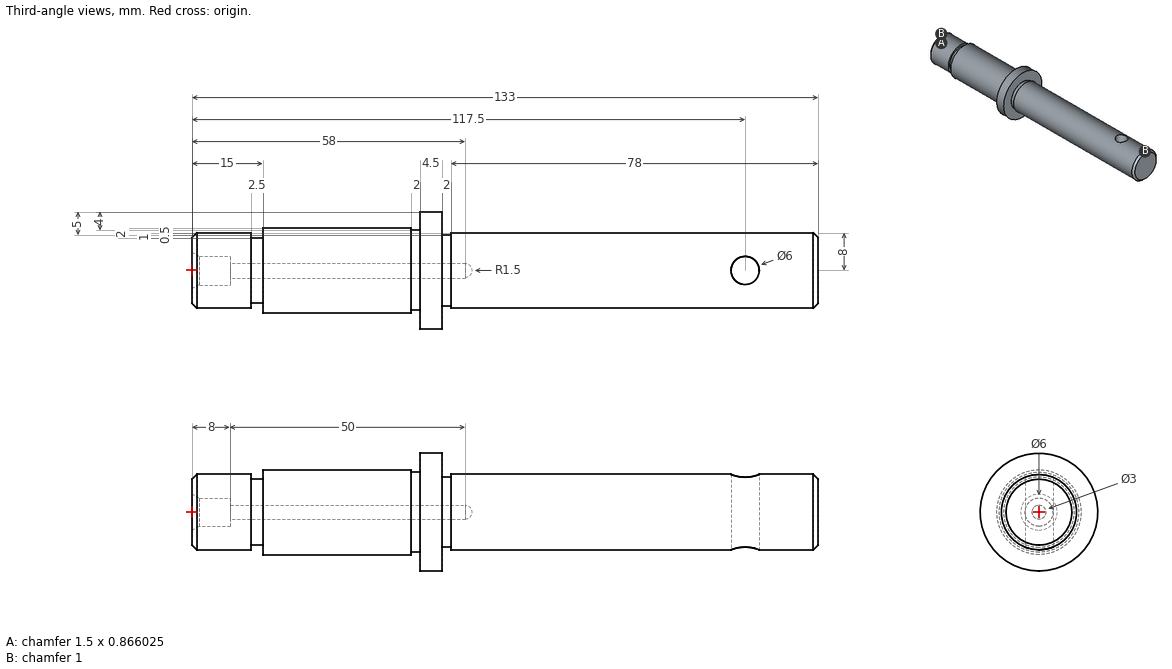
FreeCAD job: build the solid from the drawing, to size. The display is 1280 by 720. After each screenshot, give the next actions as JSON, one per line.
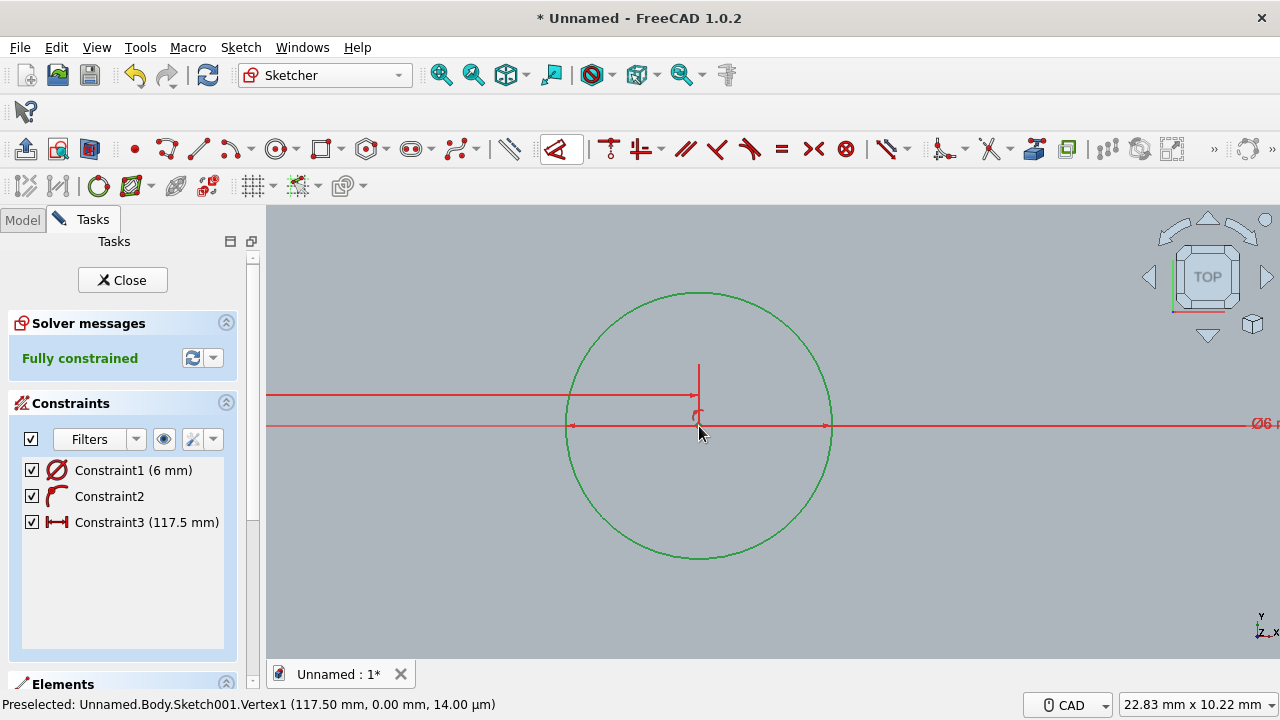
{"action": "left_click", "coordinate": [123, 280]}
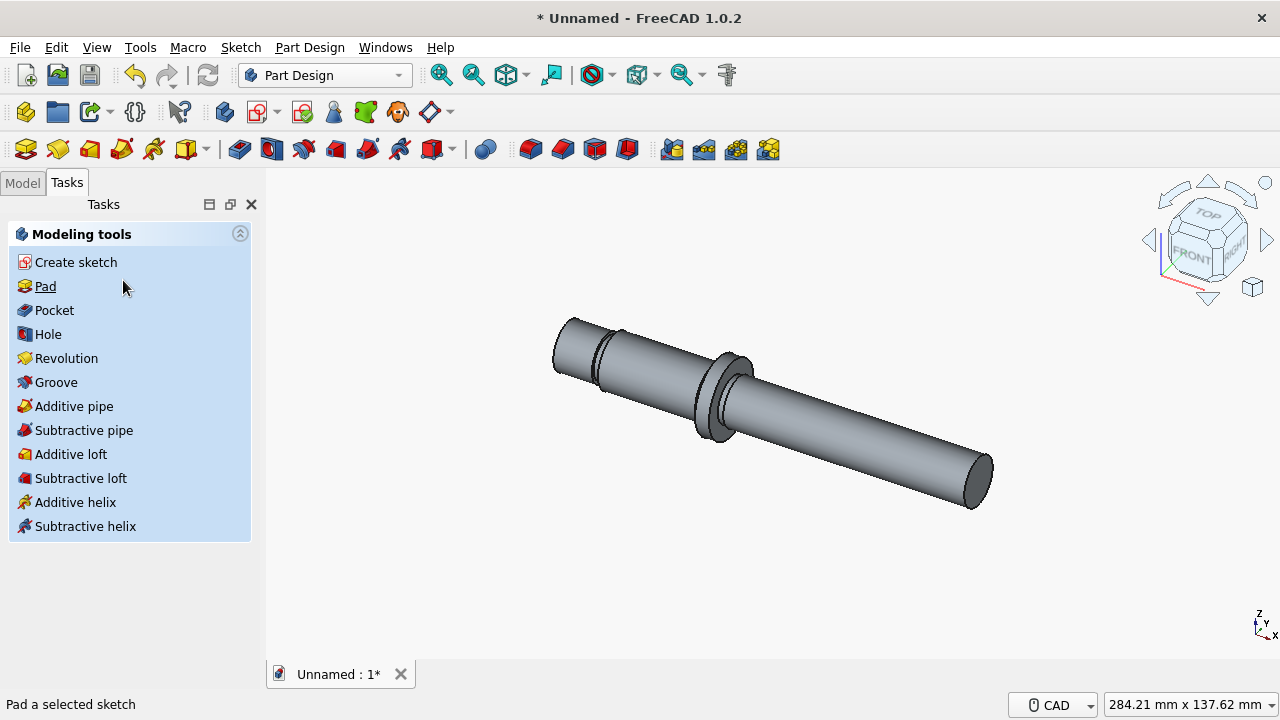
{"action": "left_click", "coordinate": [240, 150]}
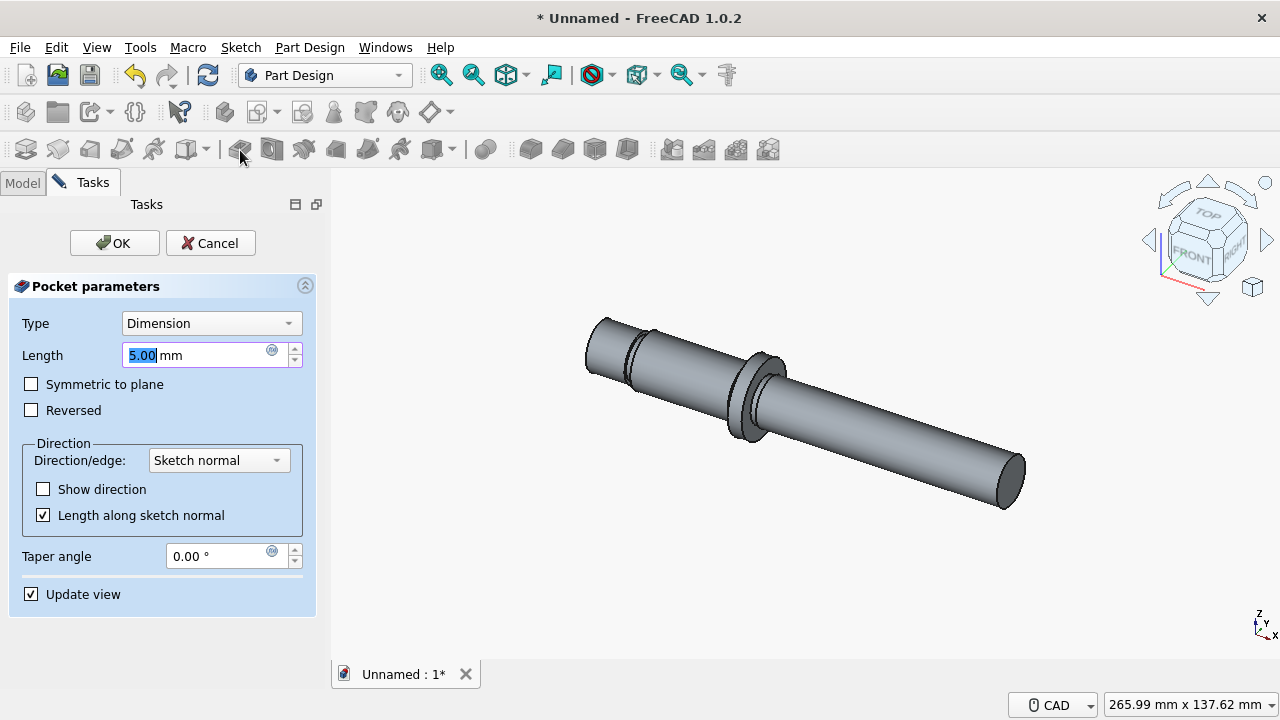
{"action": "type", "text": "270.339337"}
{"action": "key", "text": "Tab"}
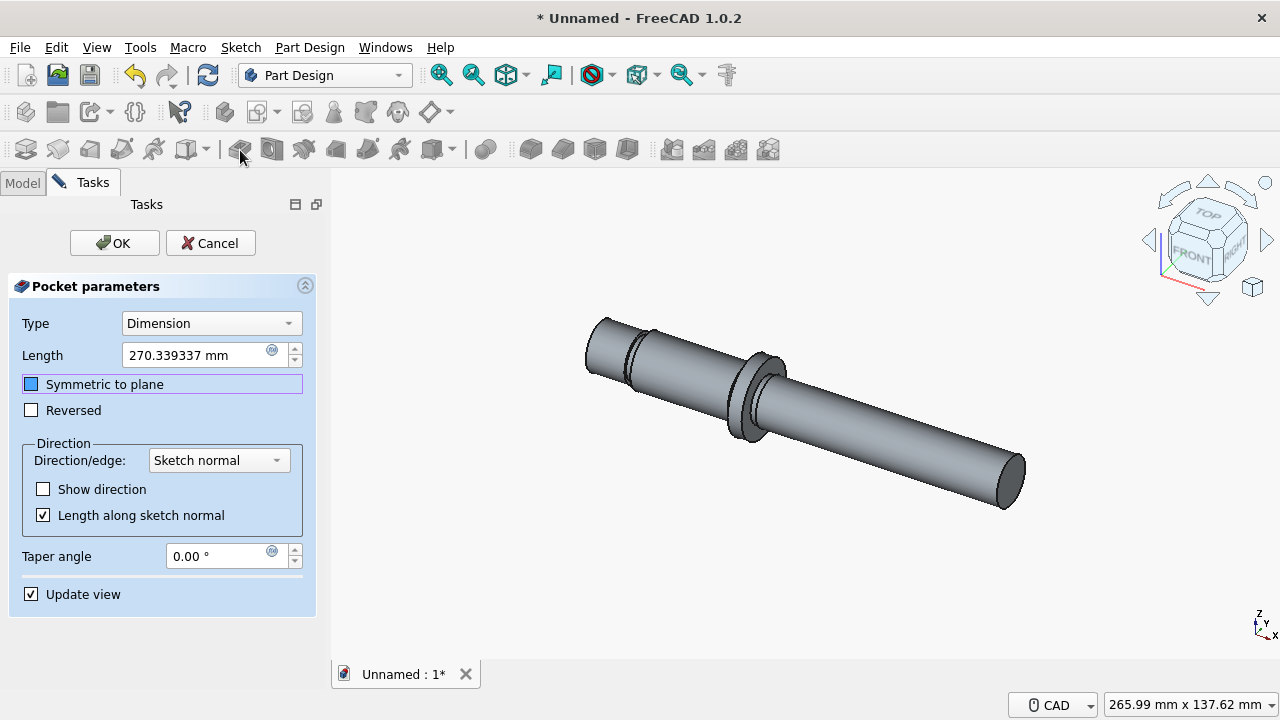
{"action": "left_click", "coordinate": [30, 384]}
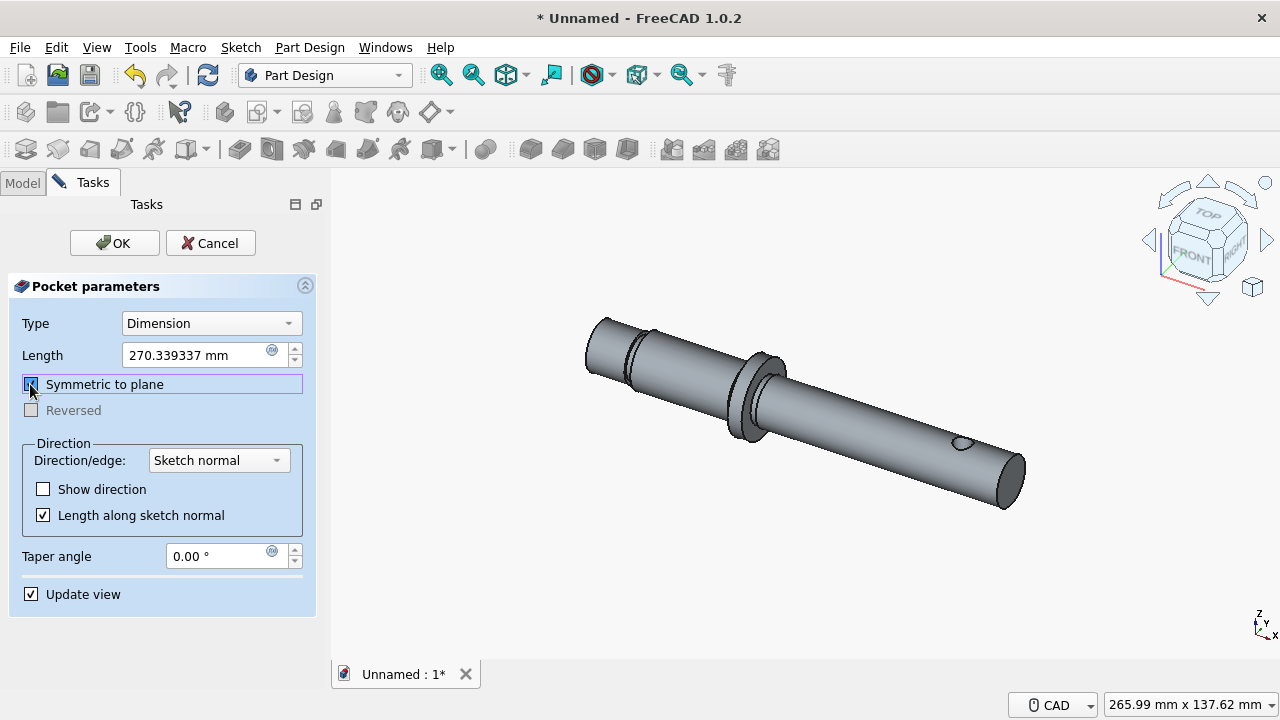
{"action": "left_click", "coordinate": [115, 243]}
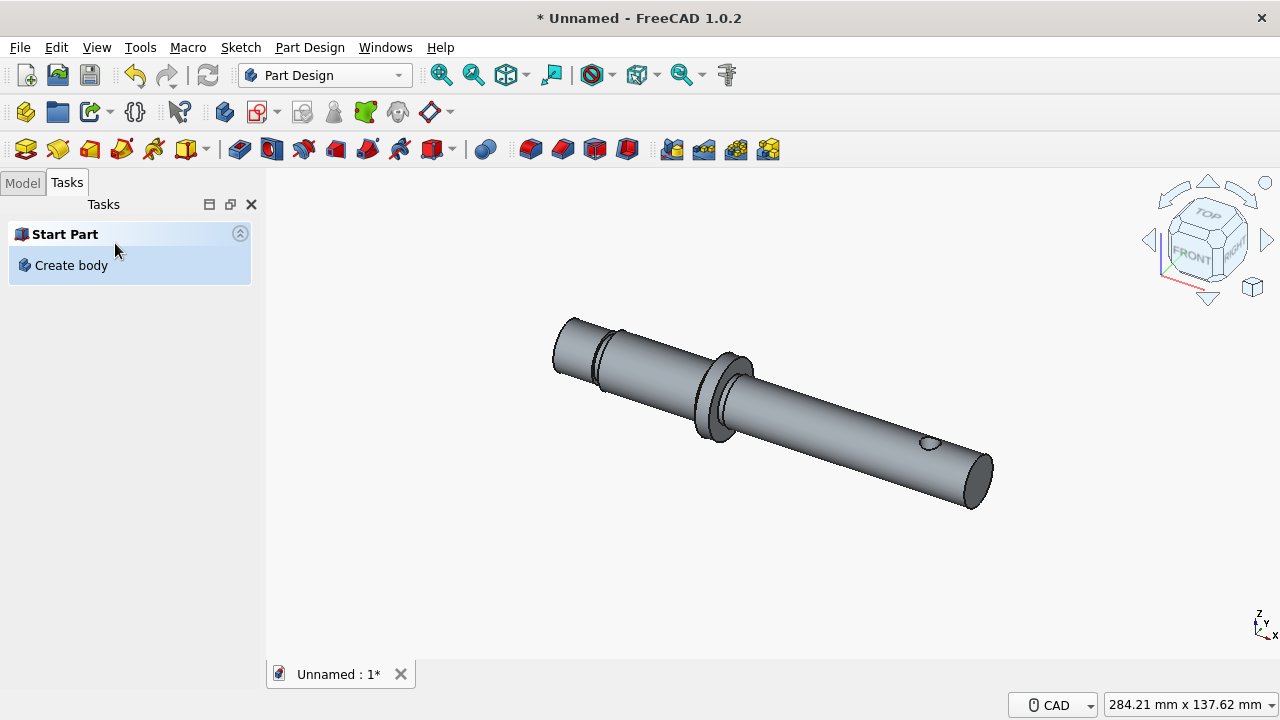
{"action": "key", "text": "6"}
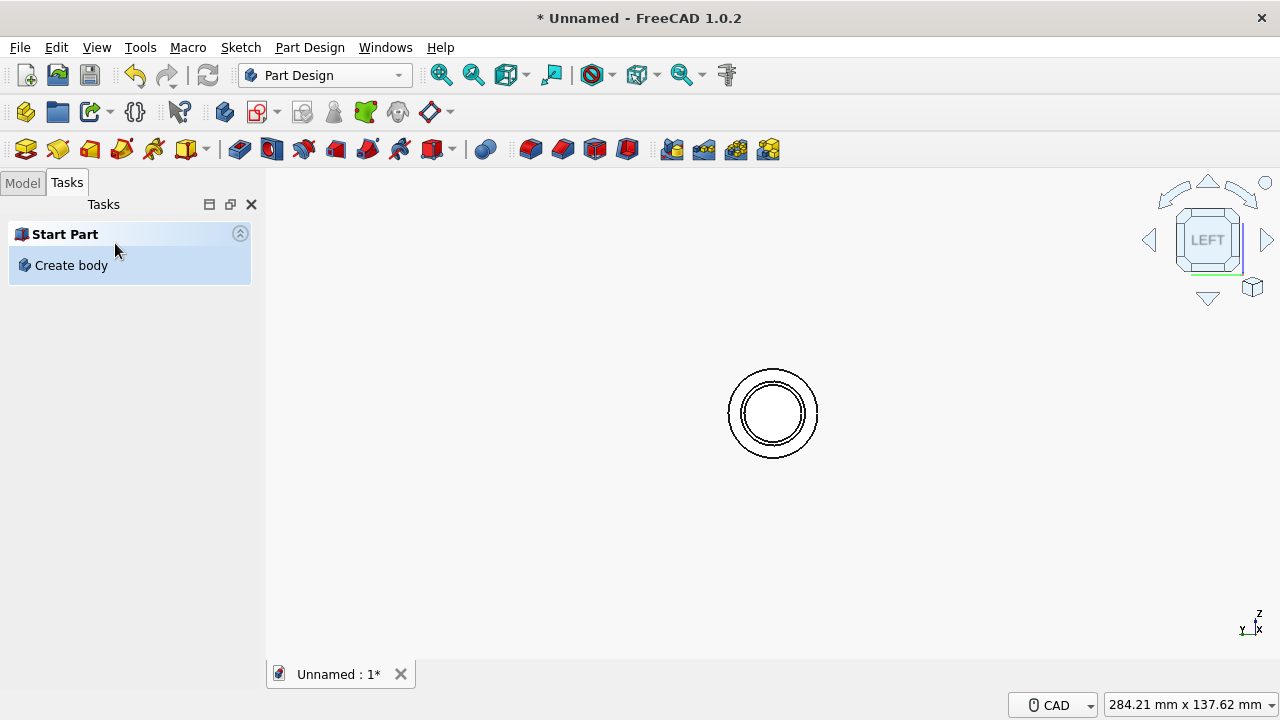
{"action": "left_click", "coordinate": [442, 76]}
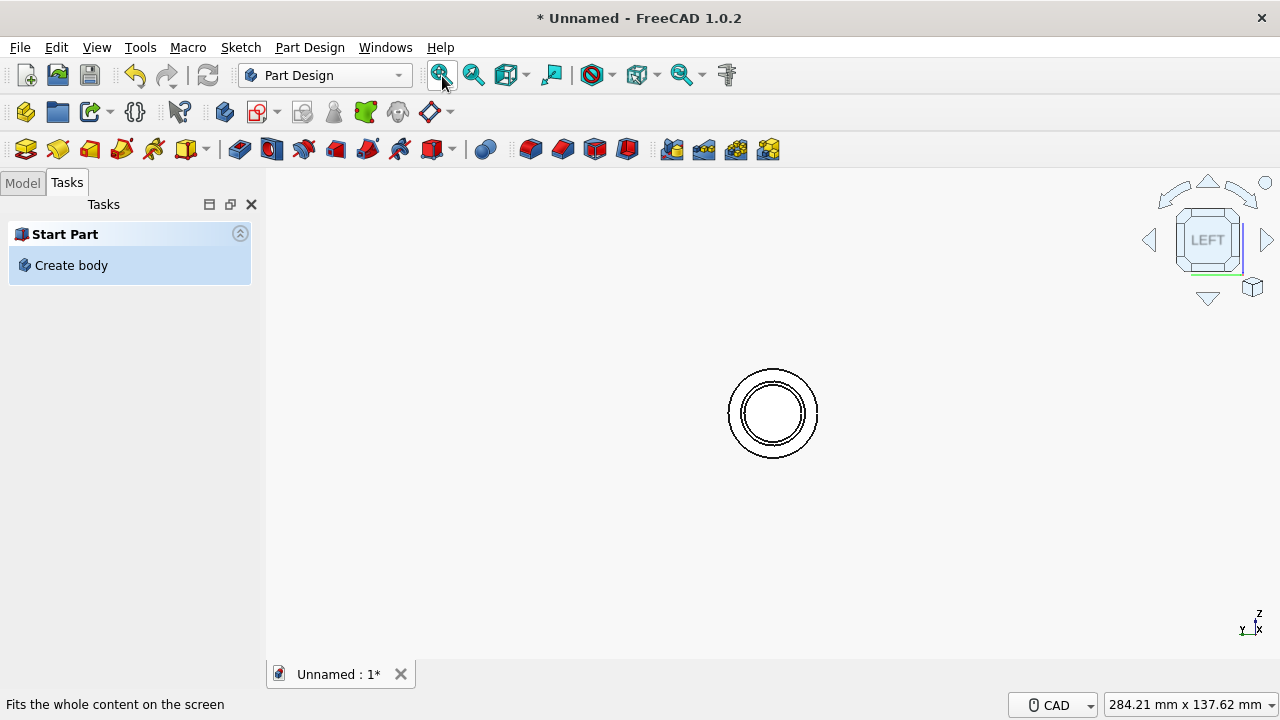
{"action": "left_click", "coordinate": [773, 412]}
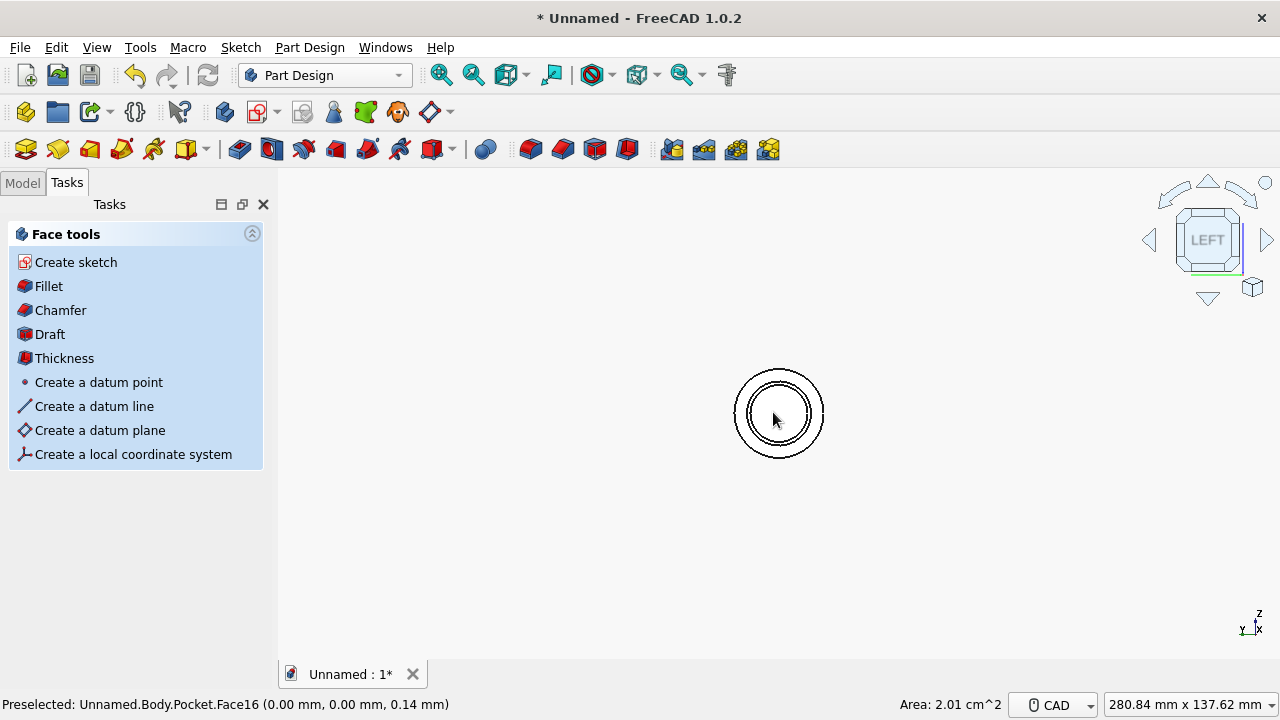
{"action": "left_click", "coordinate": [258, 112]}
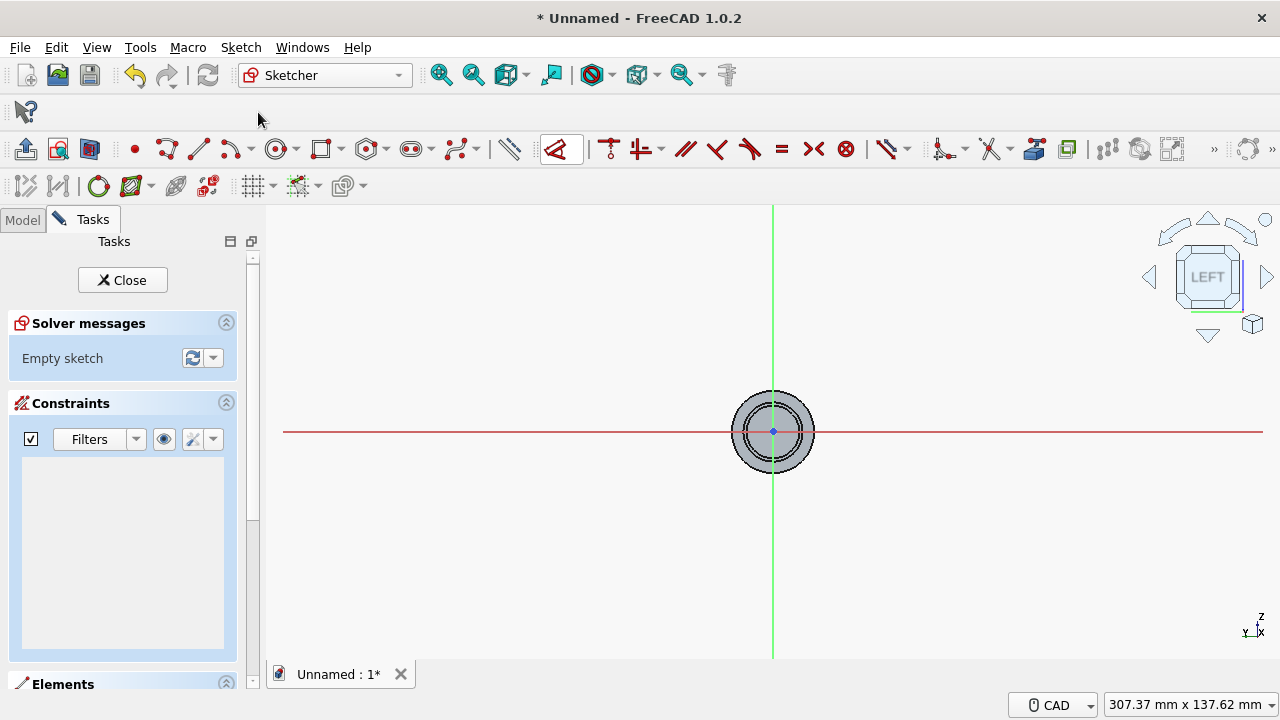
{"action": "scroll", "coordinate": [778, 432], "scroll_direction": "up", "scroll_amount": 13}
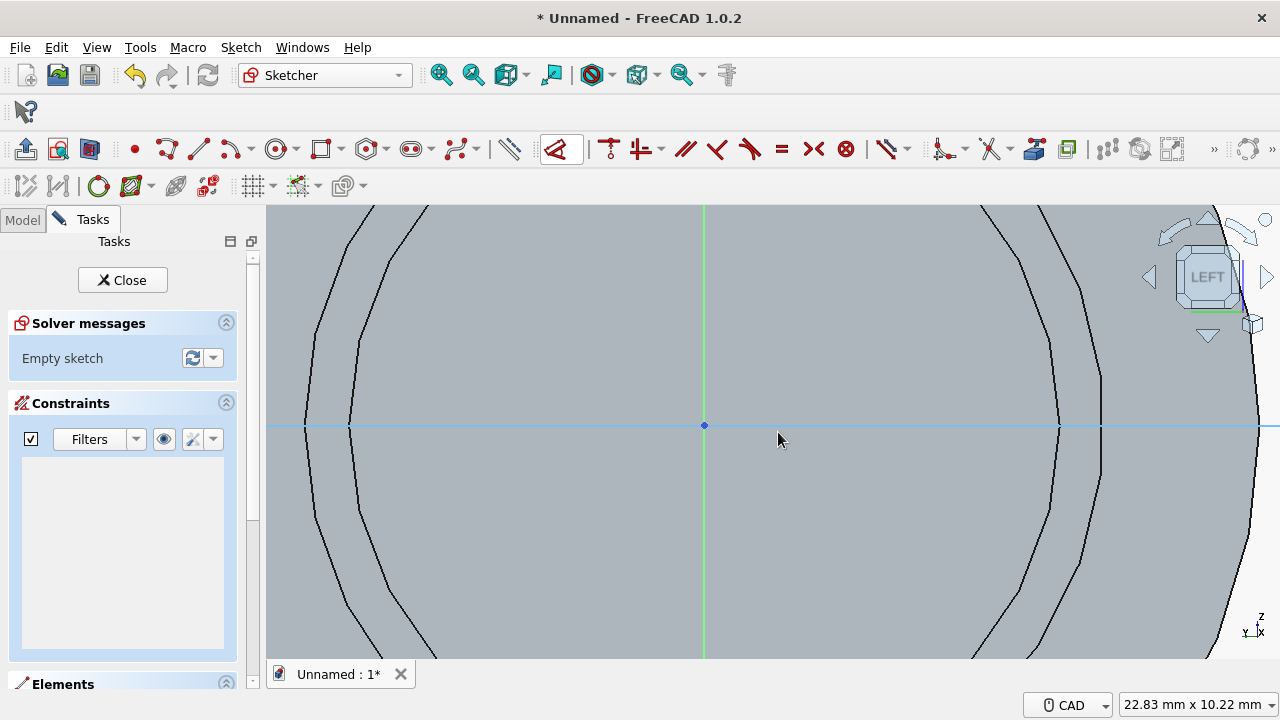
{"action": "left_click", "coordinate": [276, 150]}